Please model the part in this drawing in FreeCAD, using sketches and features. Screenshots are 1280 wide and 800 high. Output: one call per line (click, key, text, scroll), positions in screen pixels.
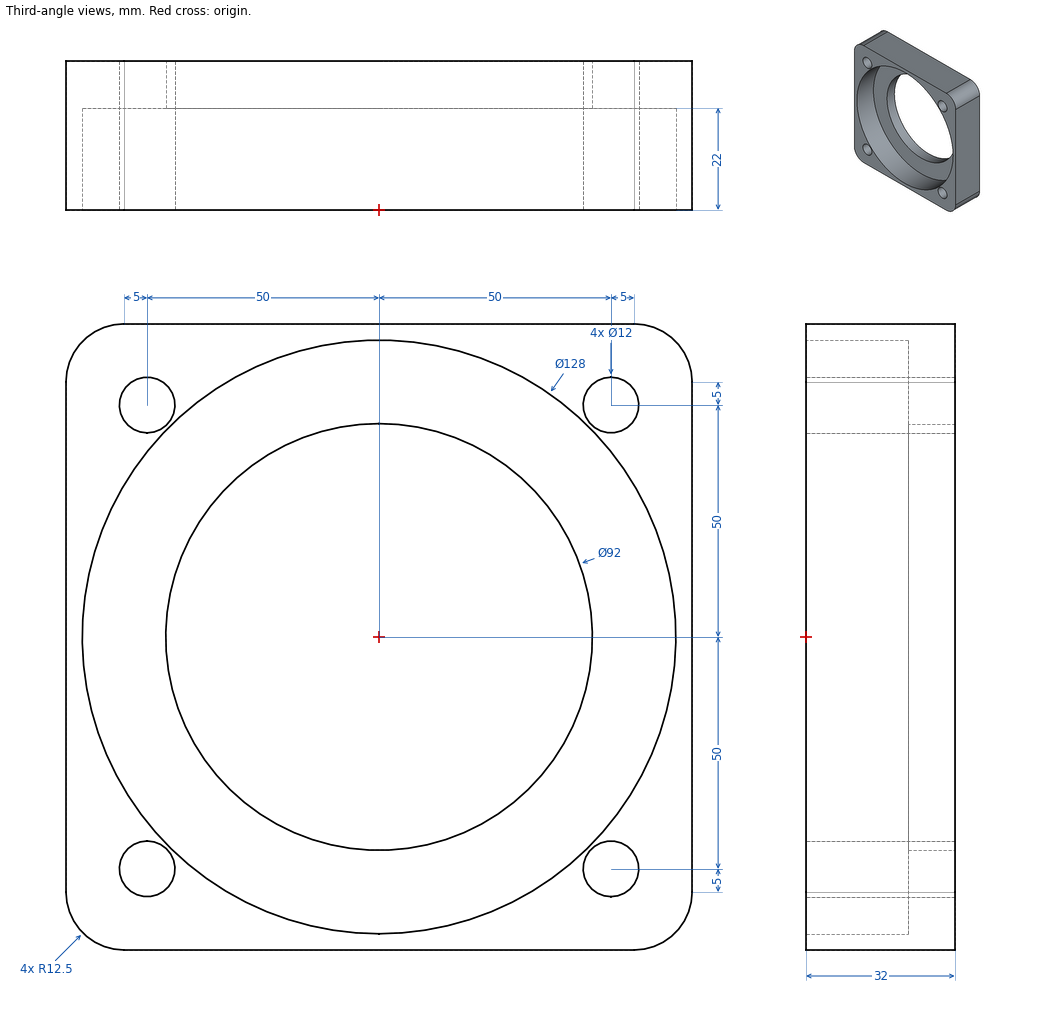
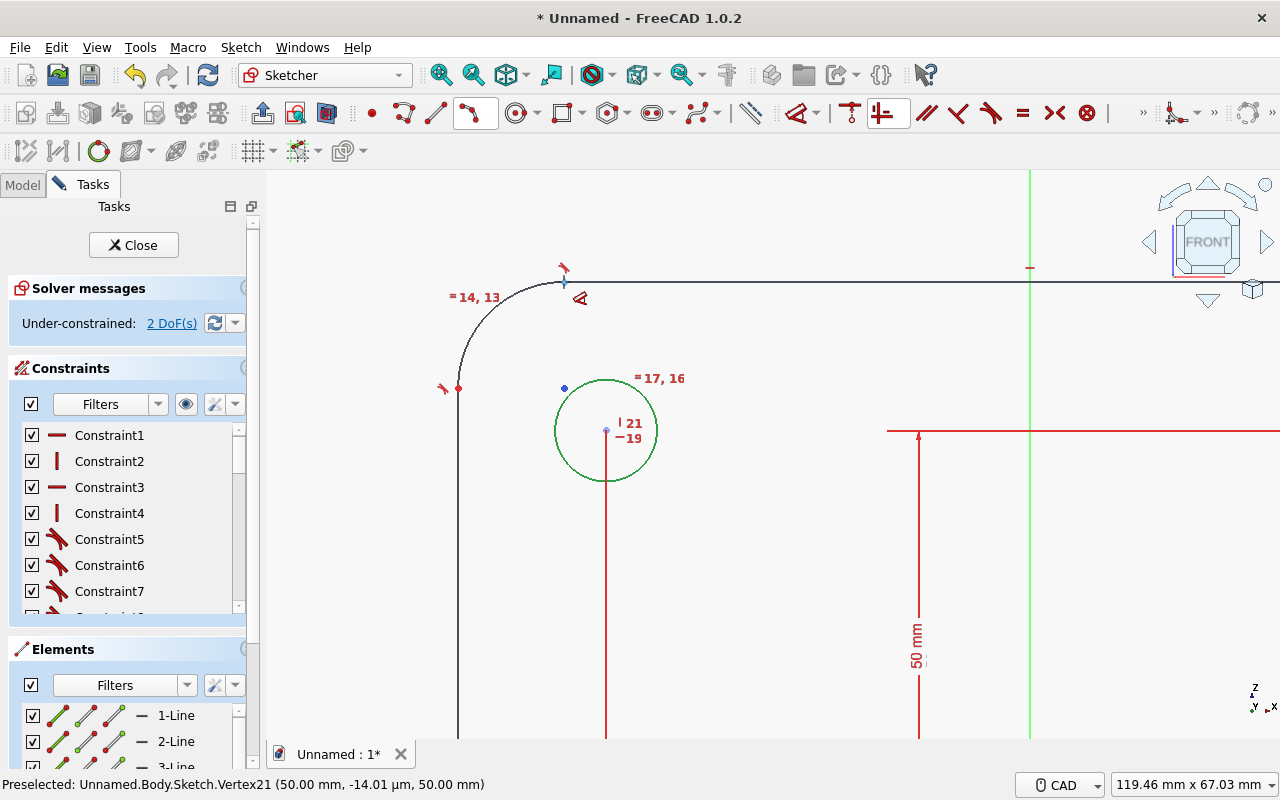
click(564, 282)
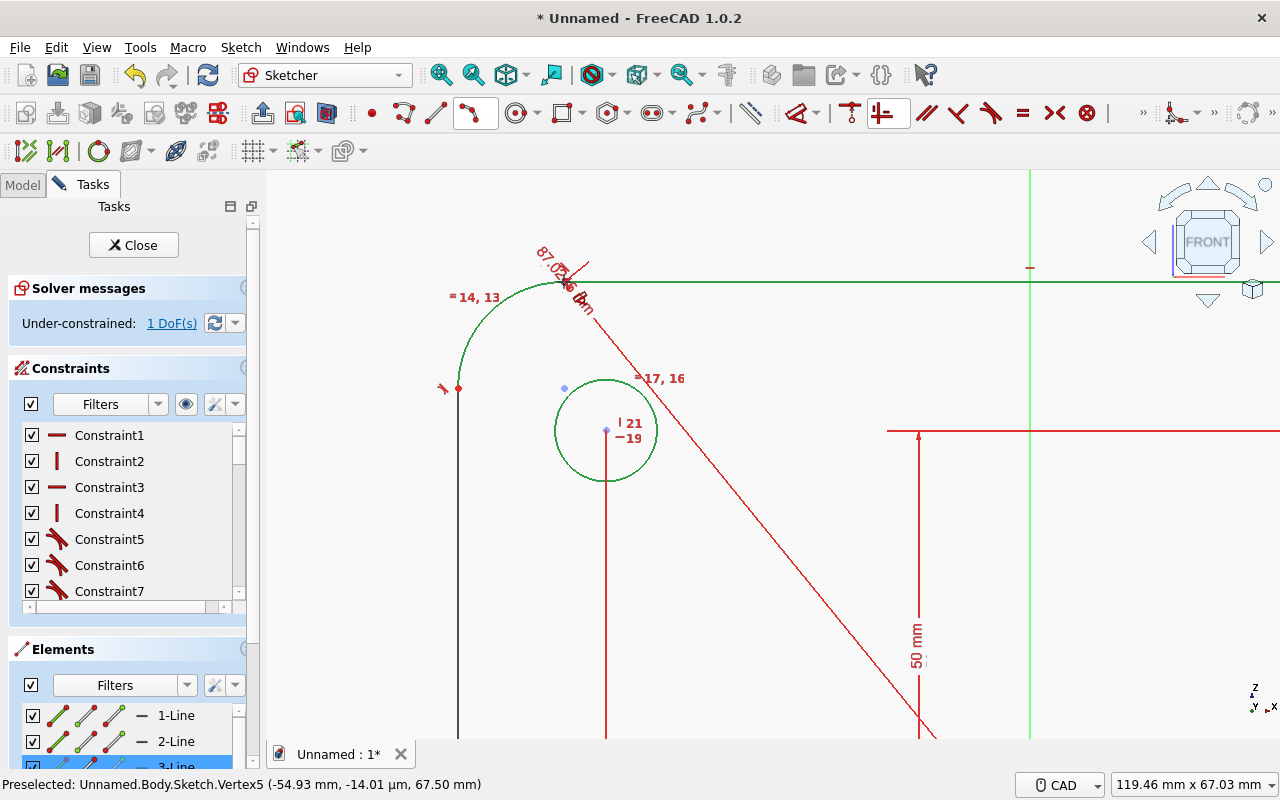
click(606, 431)
click(585, 248)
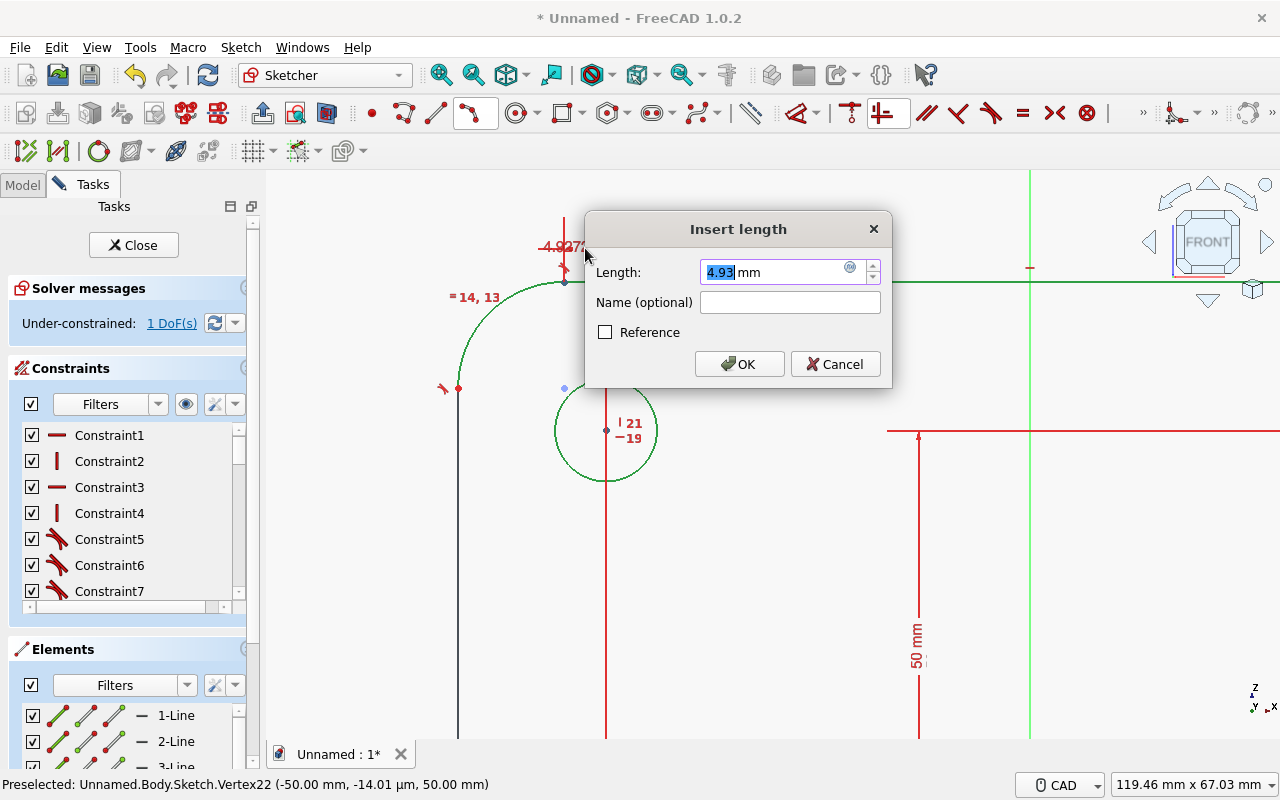
text(5)
key(Return)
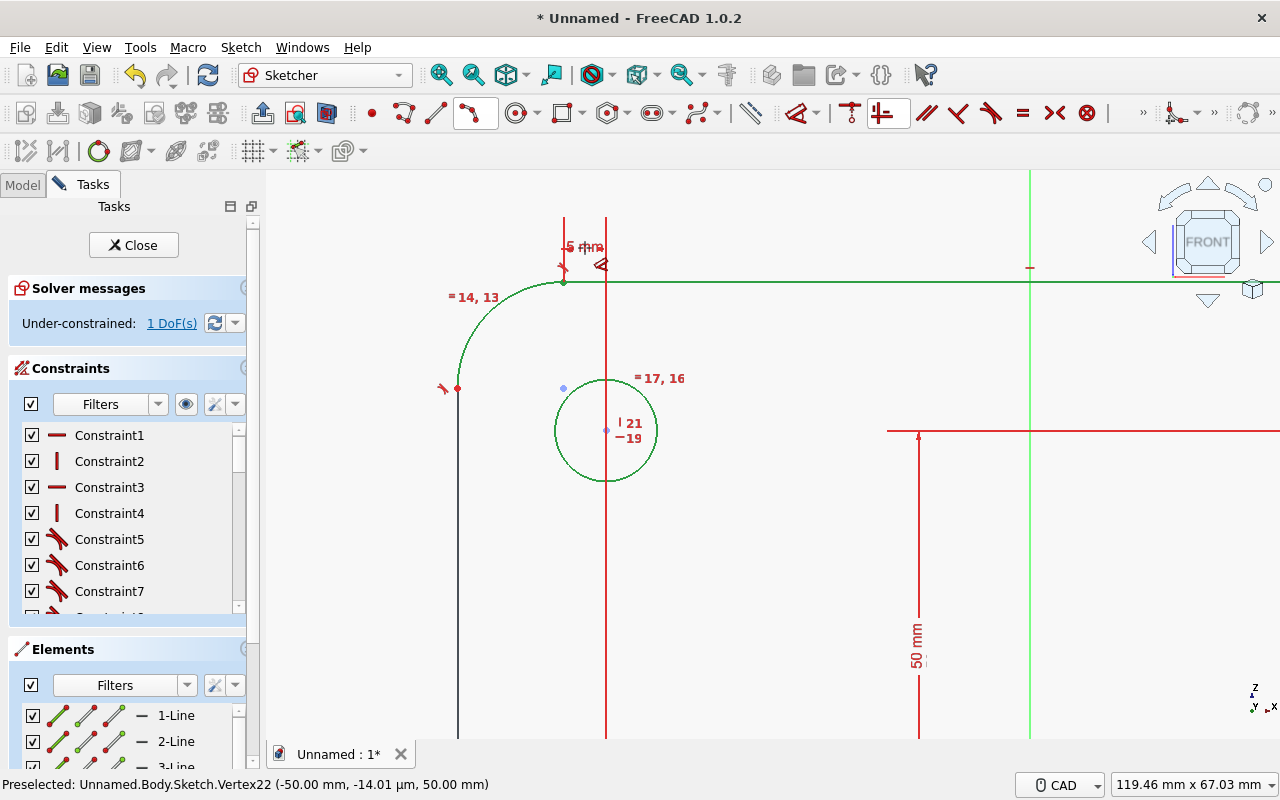
scroll(564, 282, down, 6)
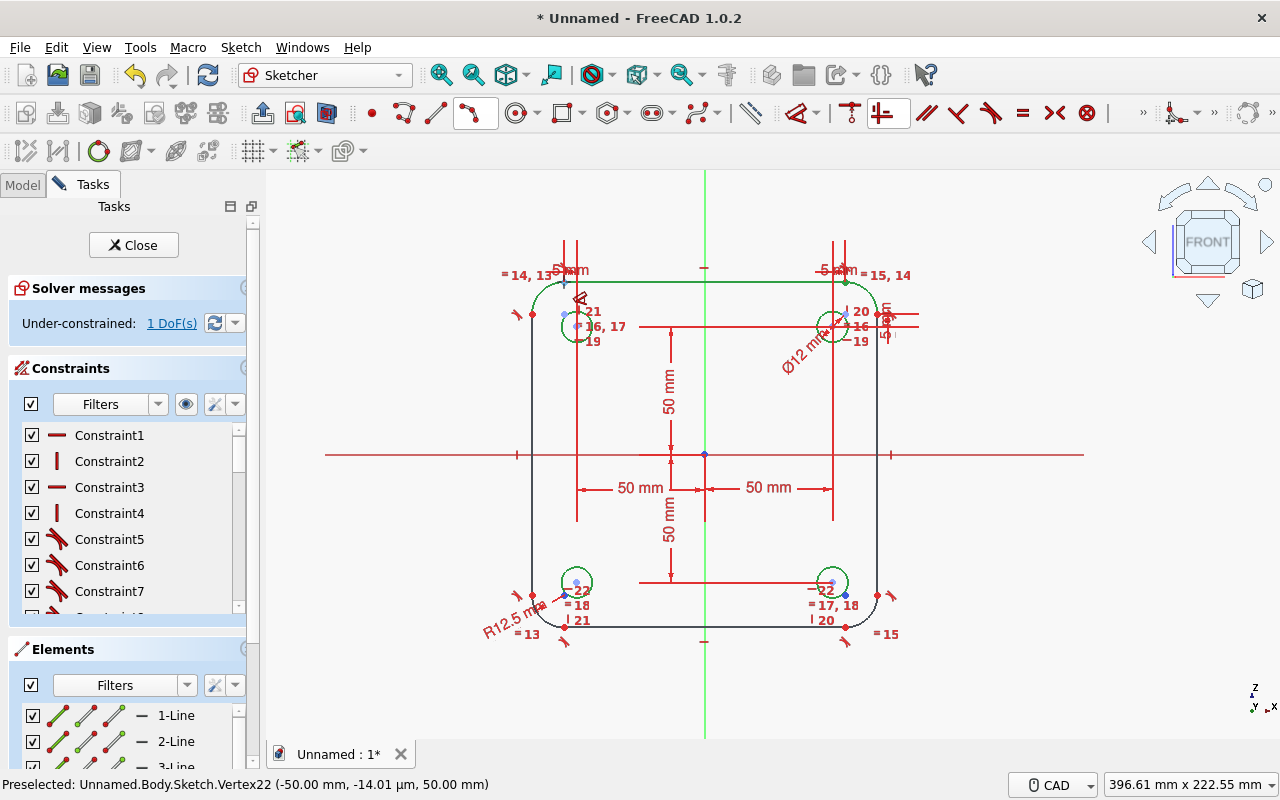
scroll(877, 596, up, 6)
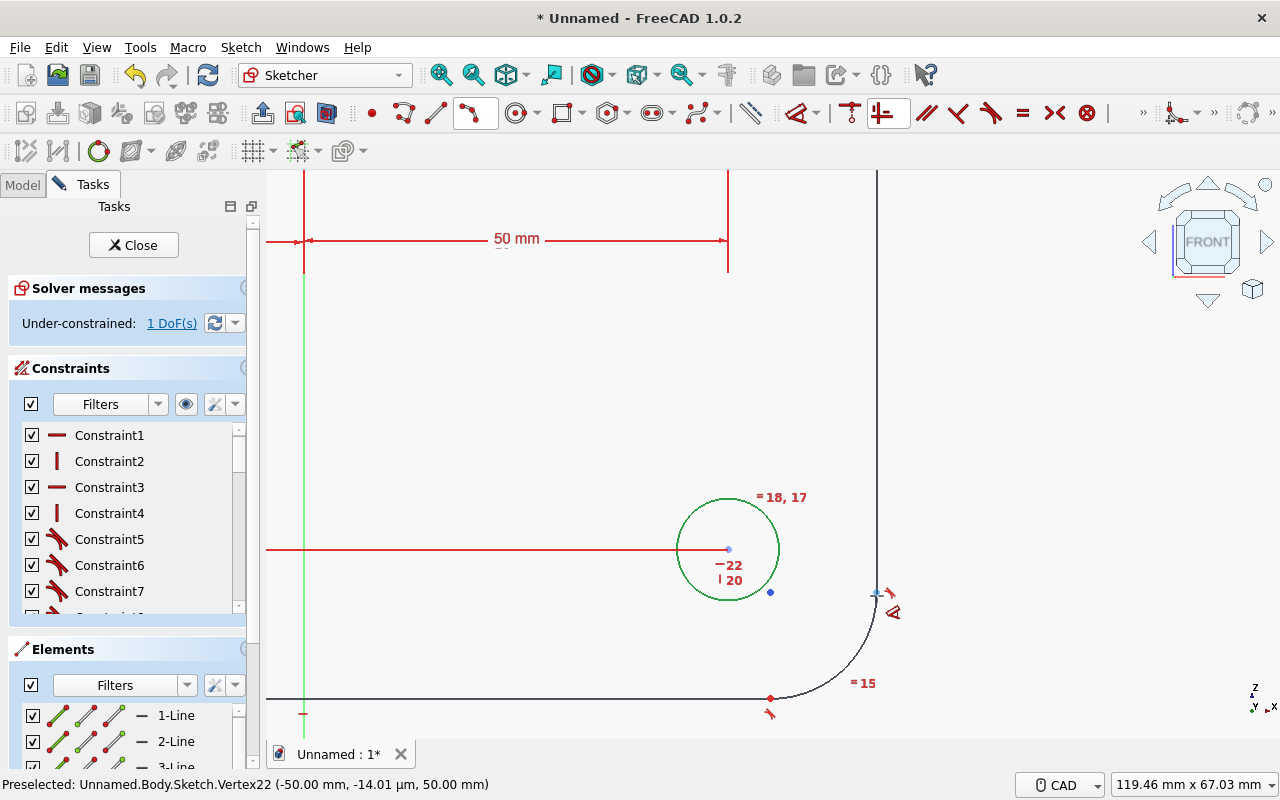
click(877, 593)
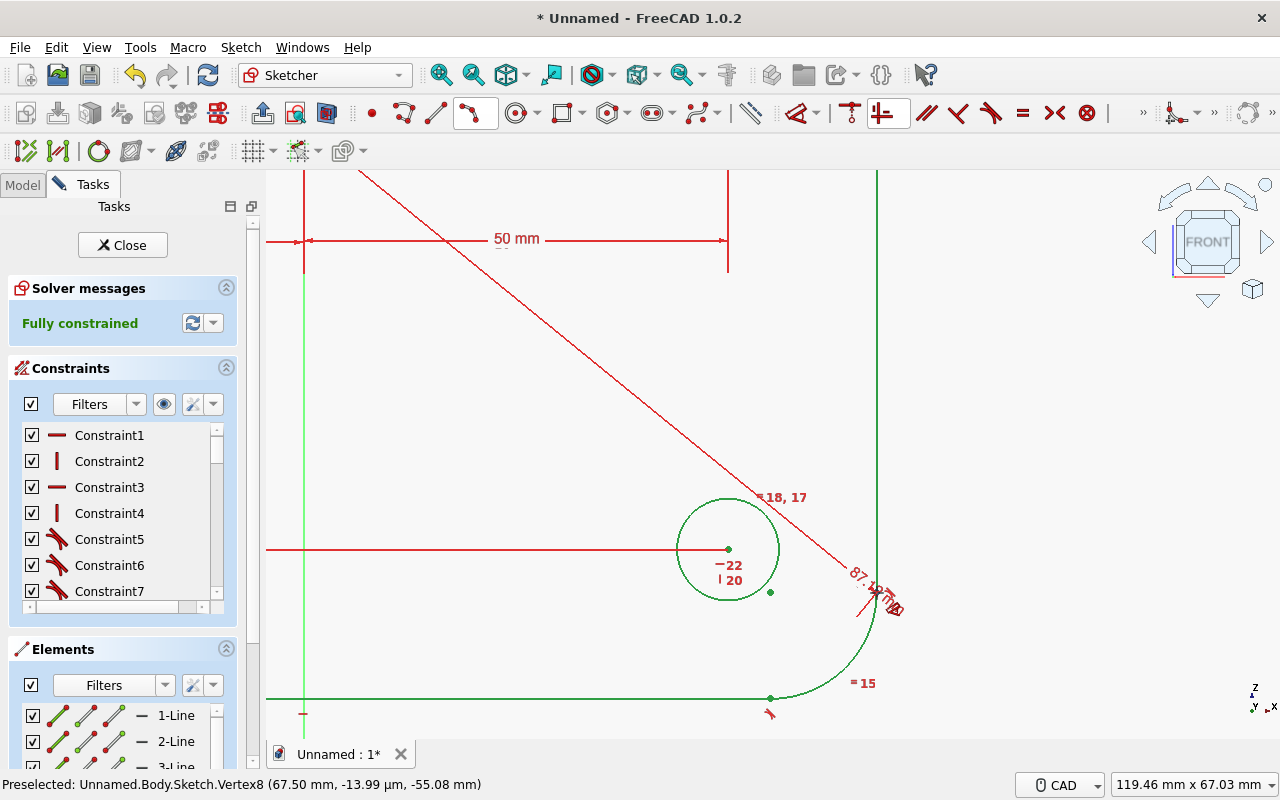
click(728, 550)
click(911, 571)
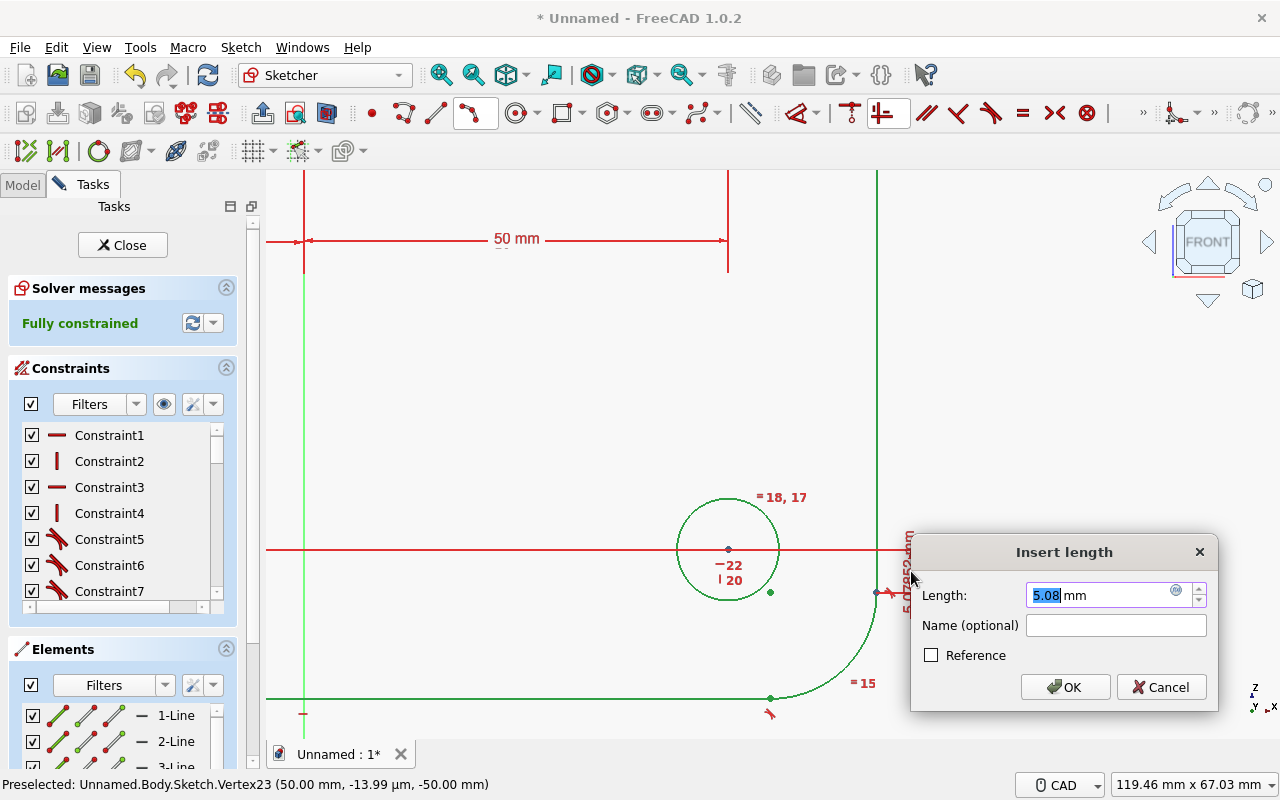
text(5)
key(Return)
key(Escape)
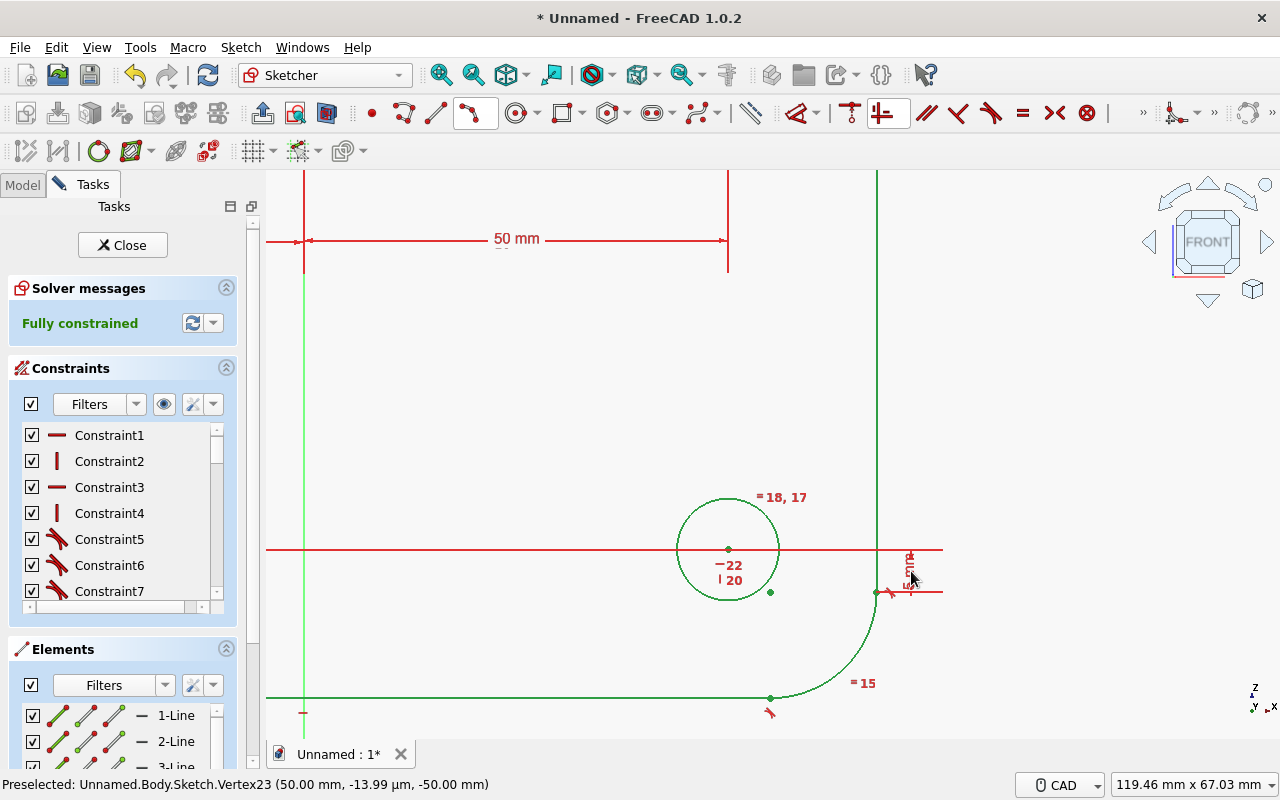
click(123, 245)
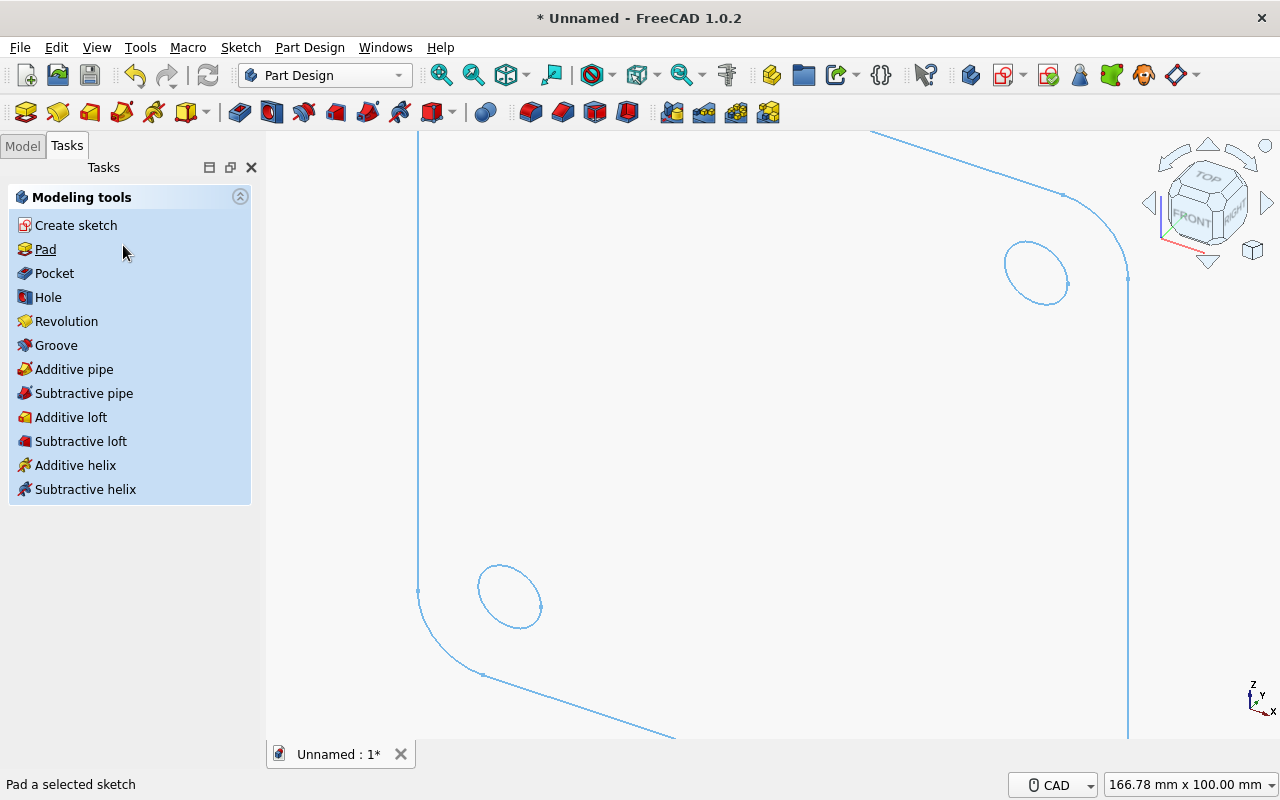
click(26, 112)